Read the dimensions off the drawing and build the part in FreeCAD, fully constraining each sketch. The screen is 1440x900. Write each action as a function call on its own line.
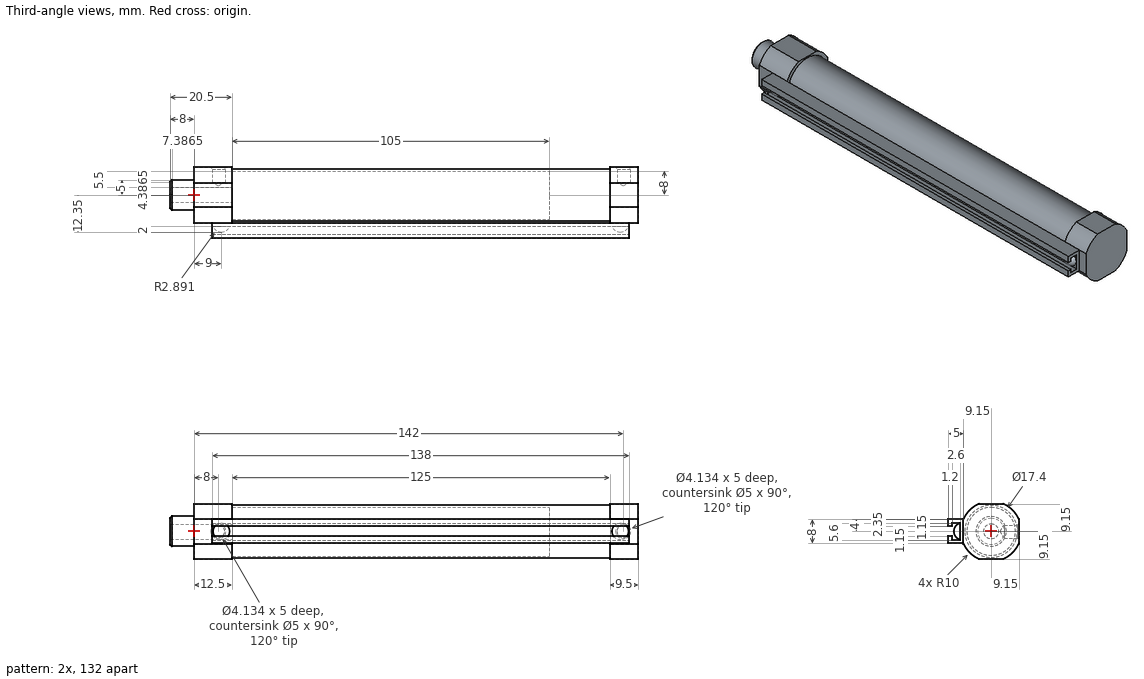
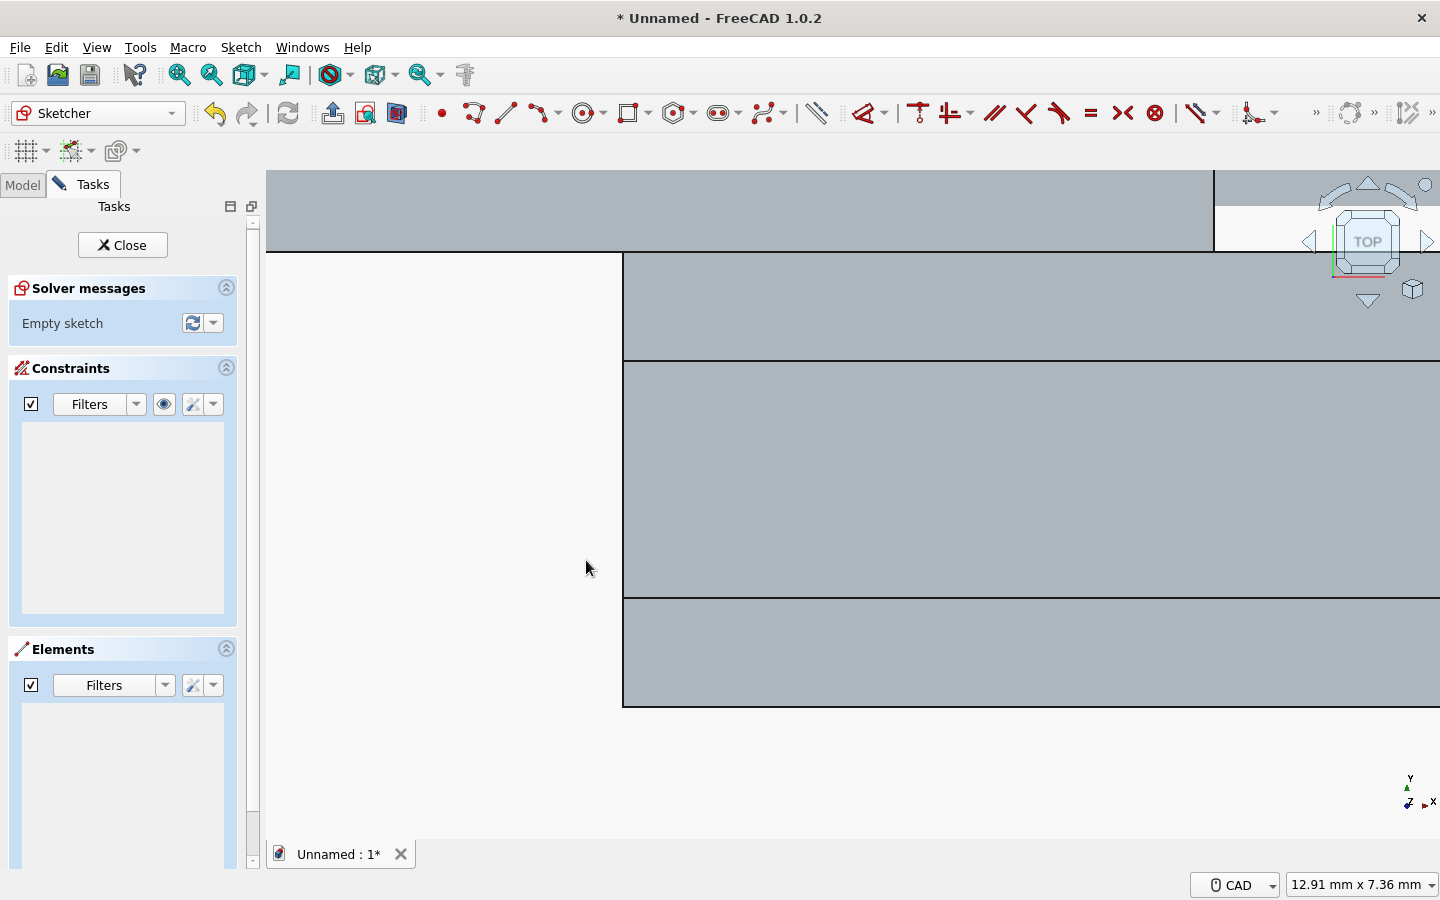
scroll(754, 470, up, 3)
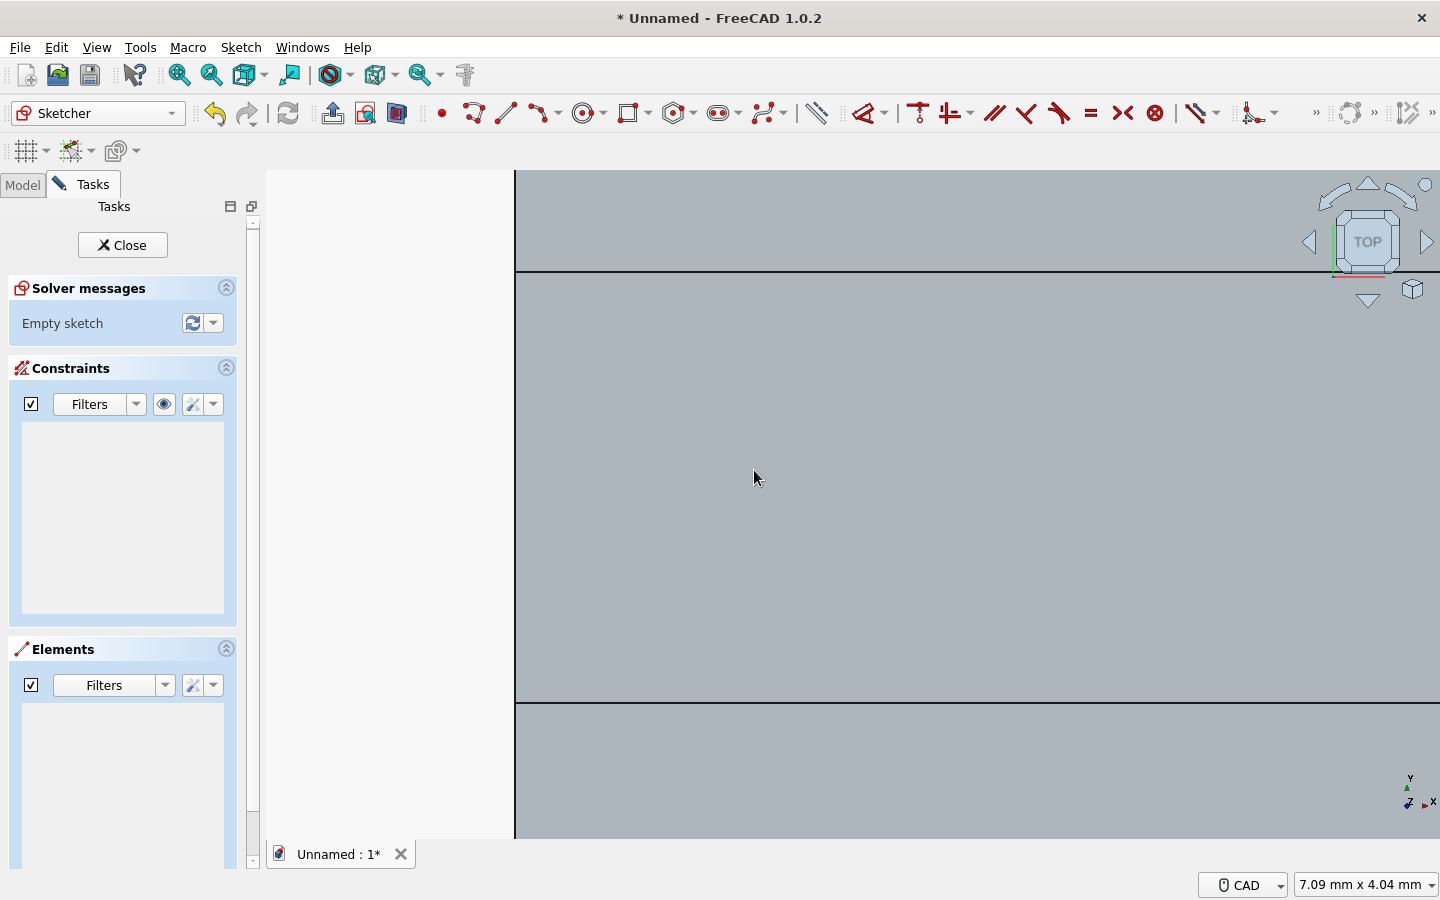
click(474, 114)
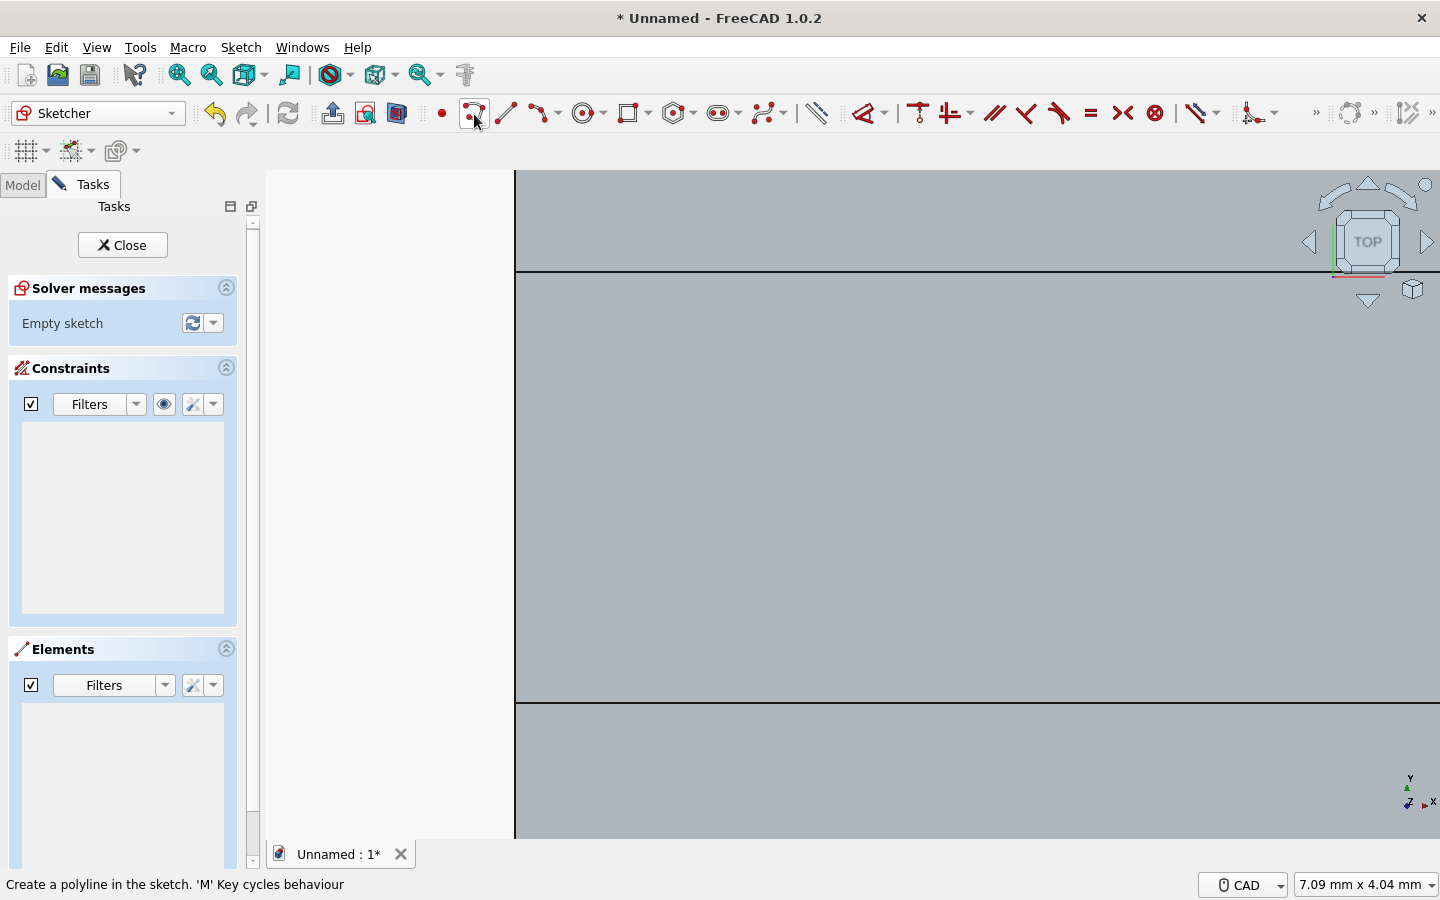
click(1012, 603)
click(1012, 272)
click(557, 272)
right_click(557, 272)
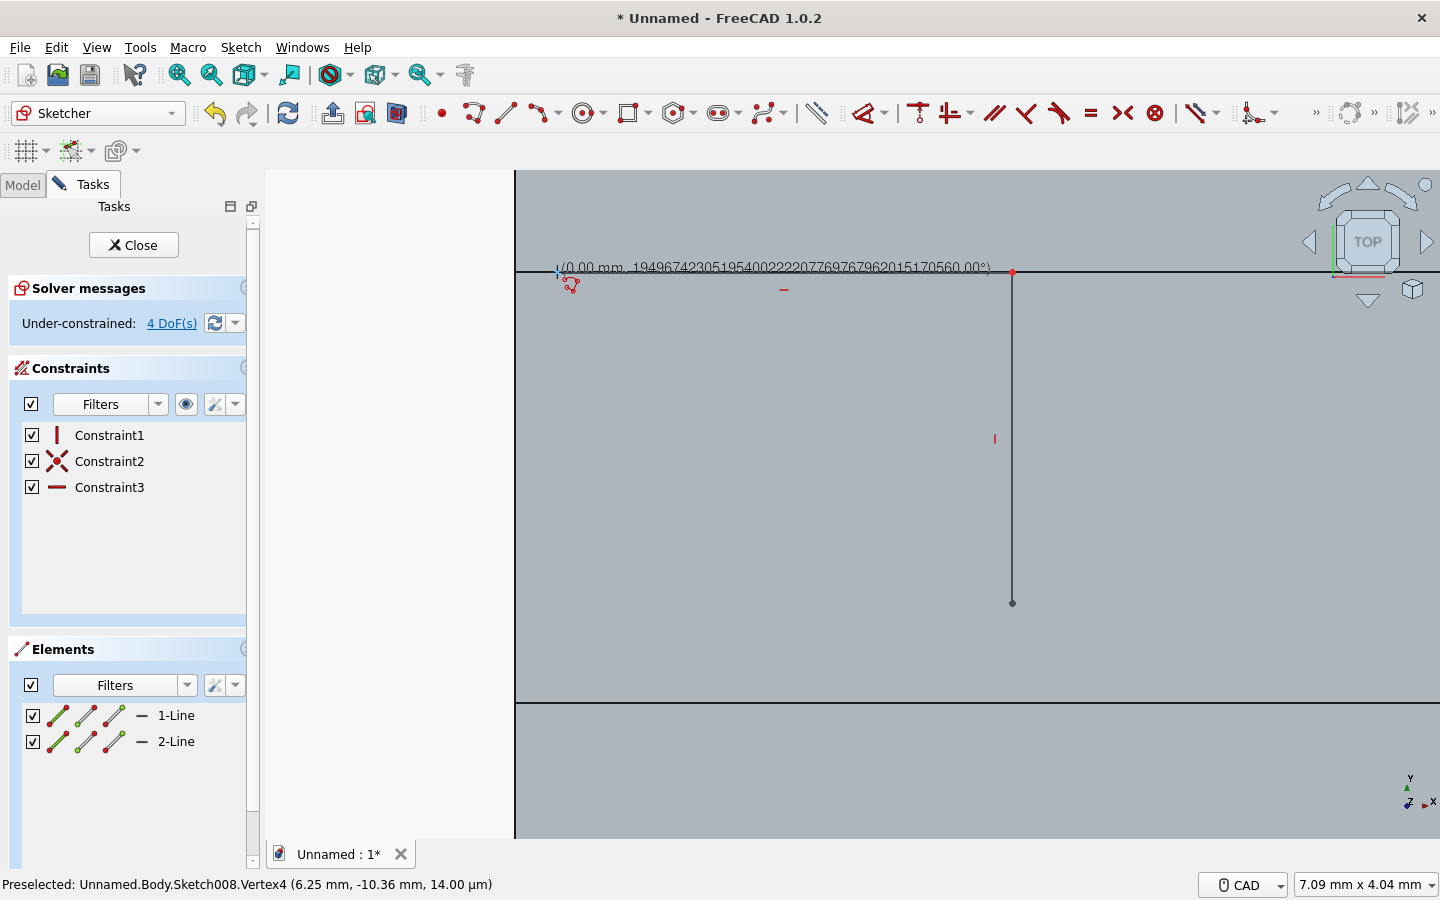
click(538, 114)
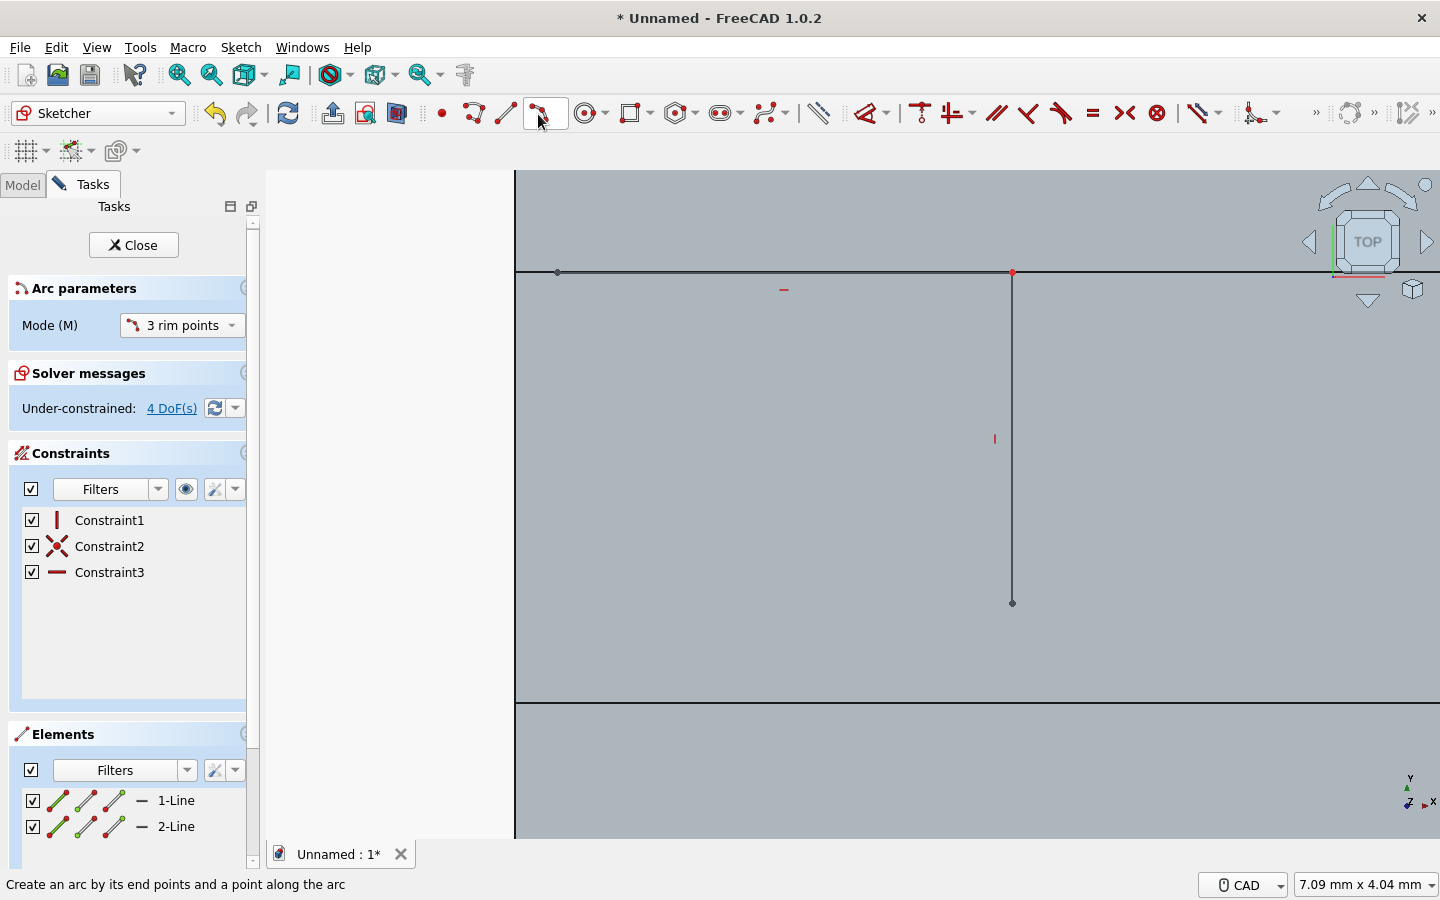
click(557, 273)
click(1012, 604)
click(731, 512)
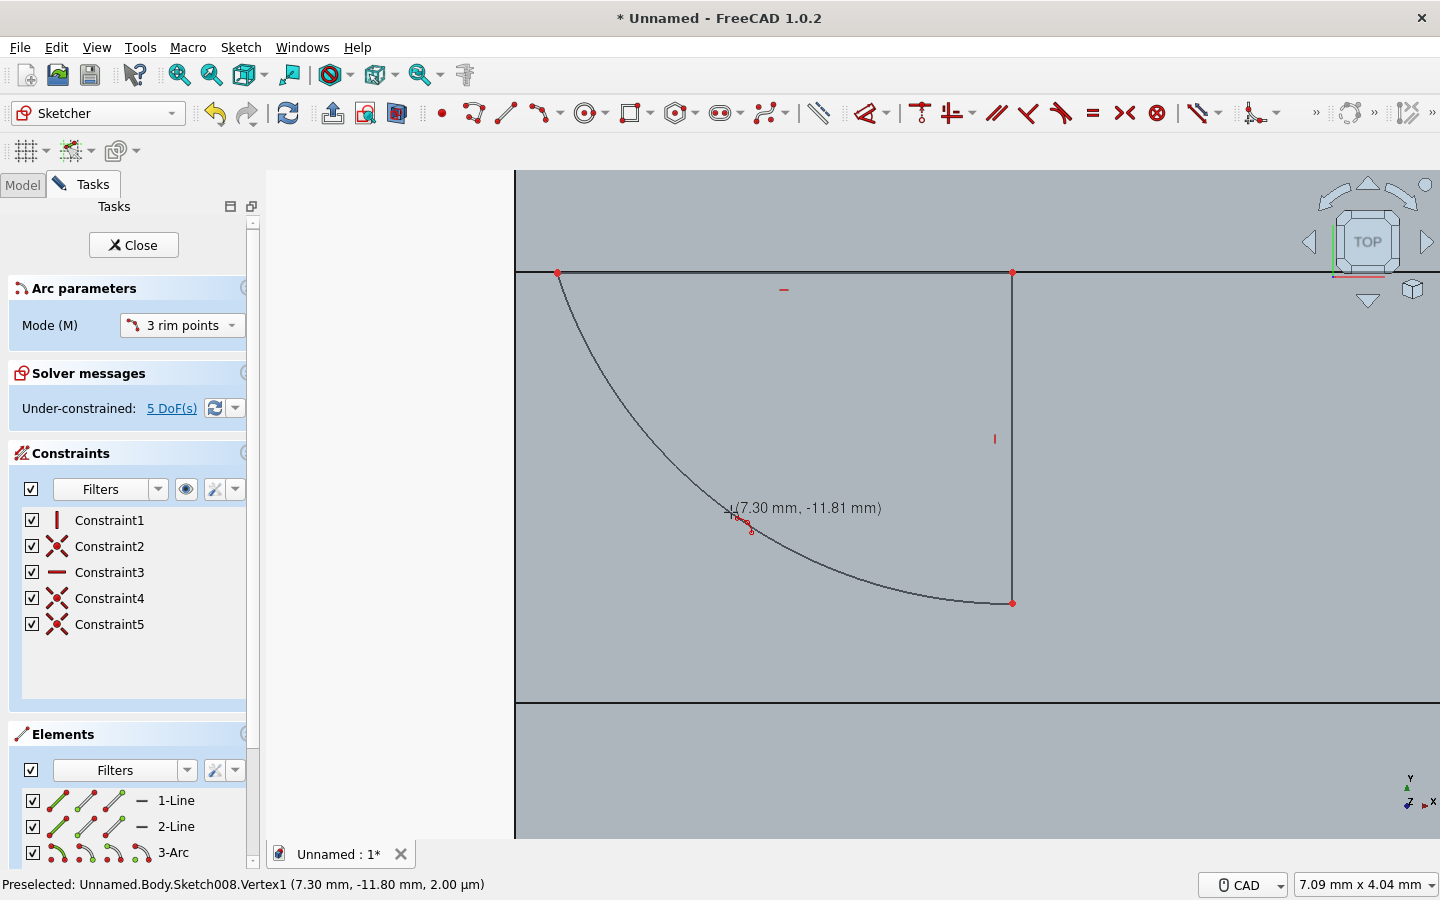
click(506, 114)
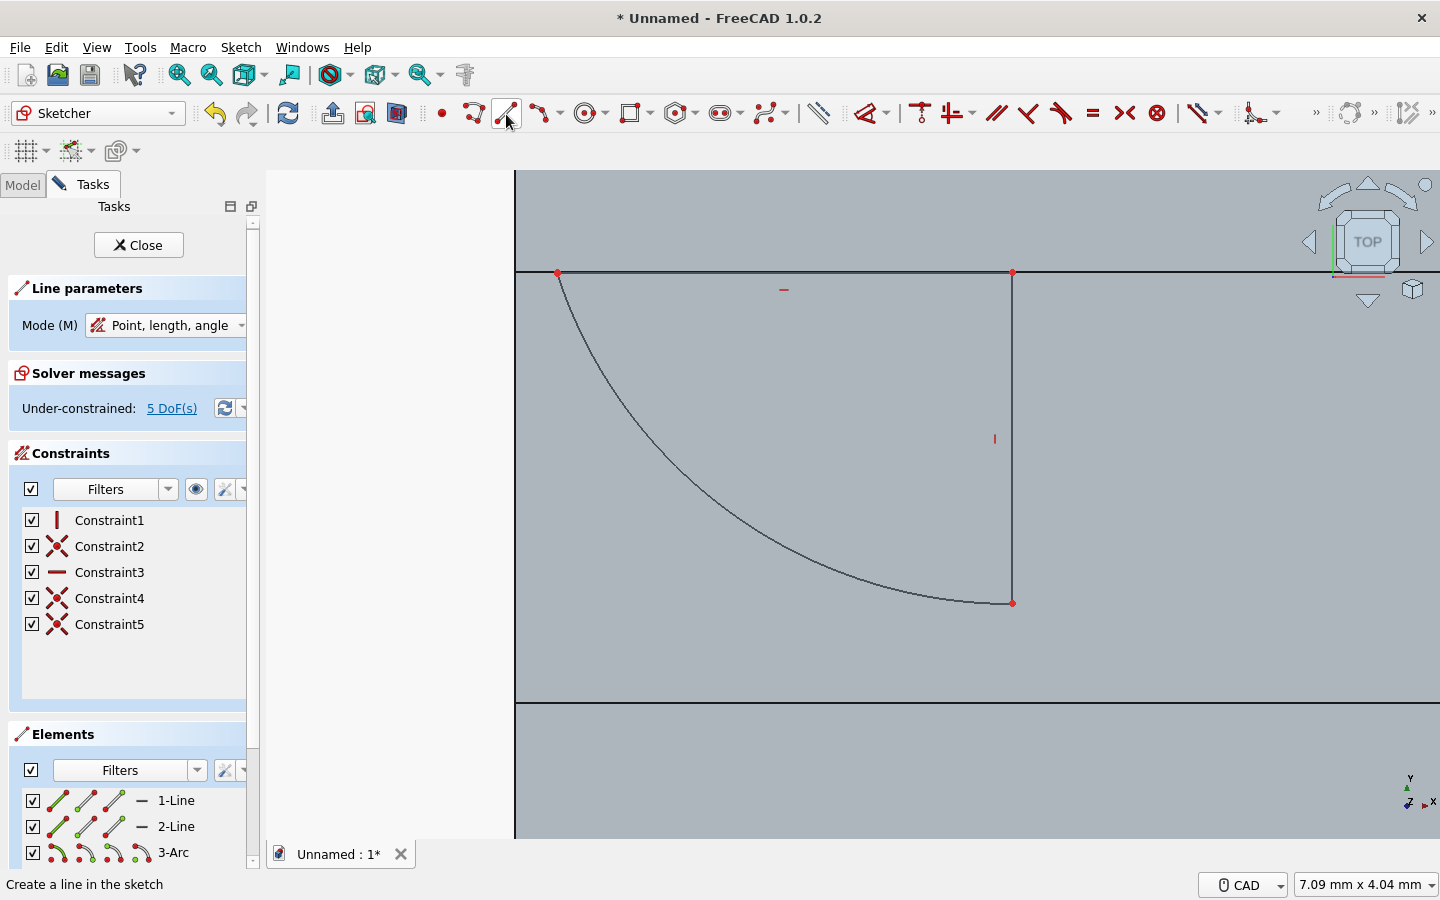
click(1012, 636)
click(1012, 736)
key(Escape)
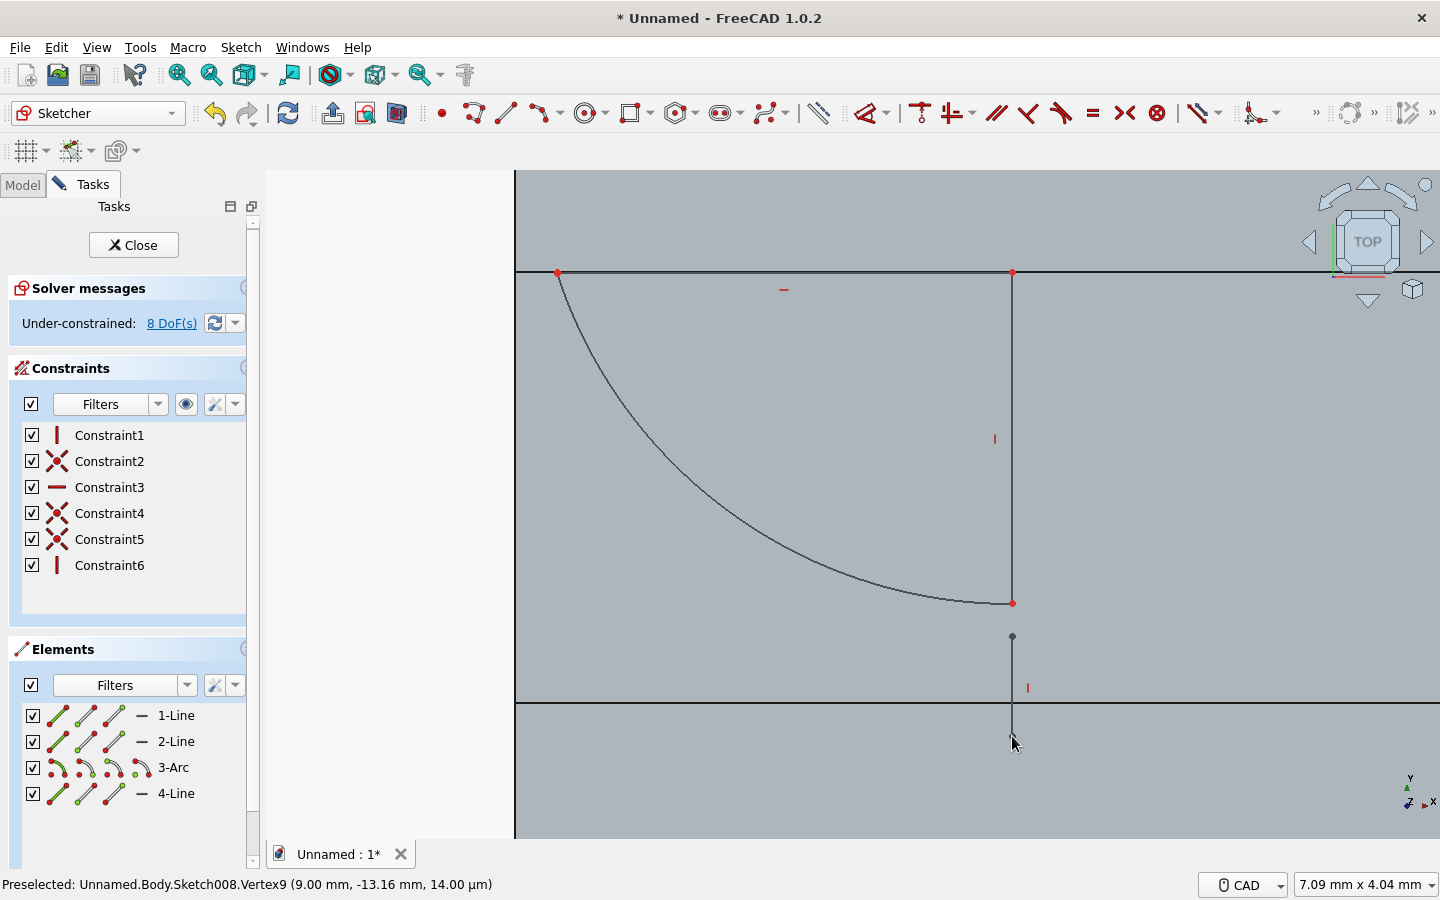
click(1012, 667)